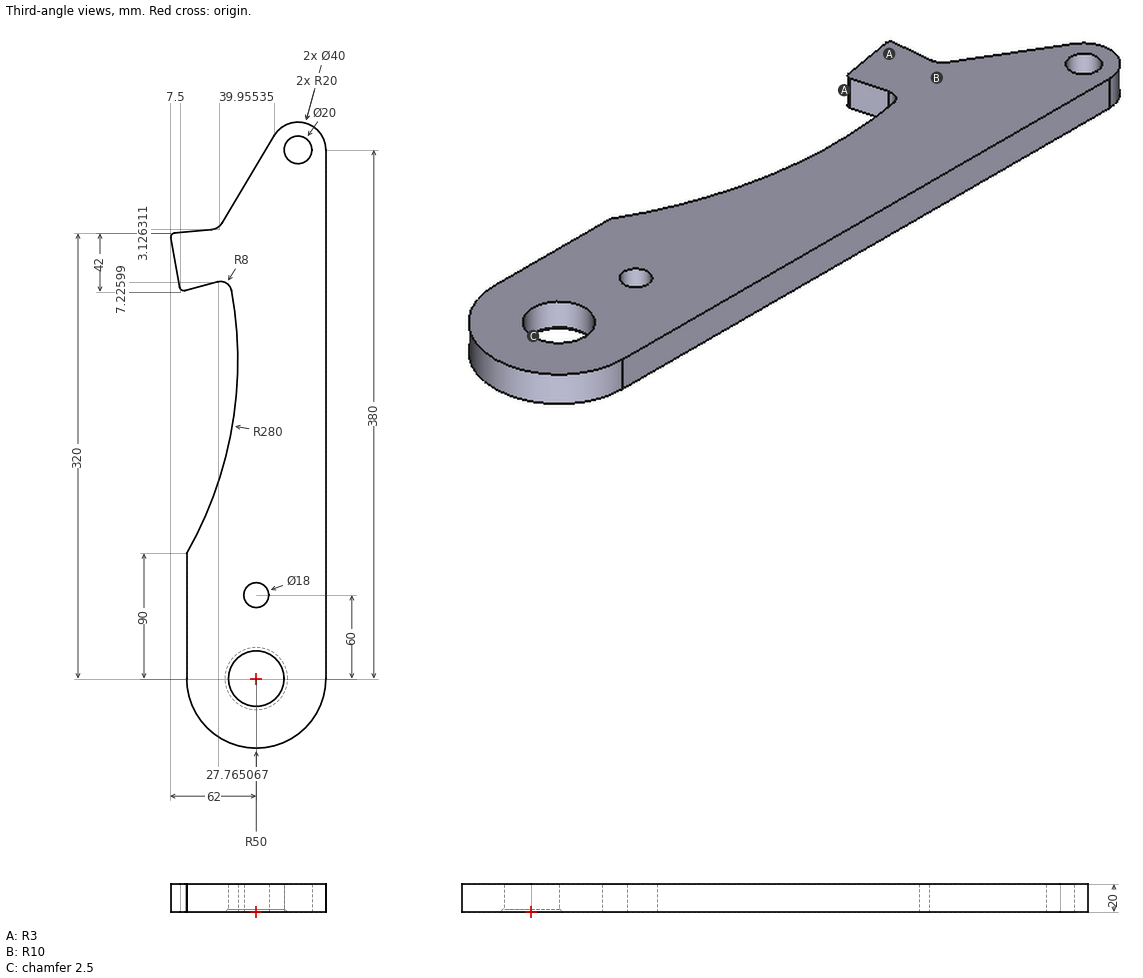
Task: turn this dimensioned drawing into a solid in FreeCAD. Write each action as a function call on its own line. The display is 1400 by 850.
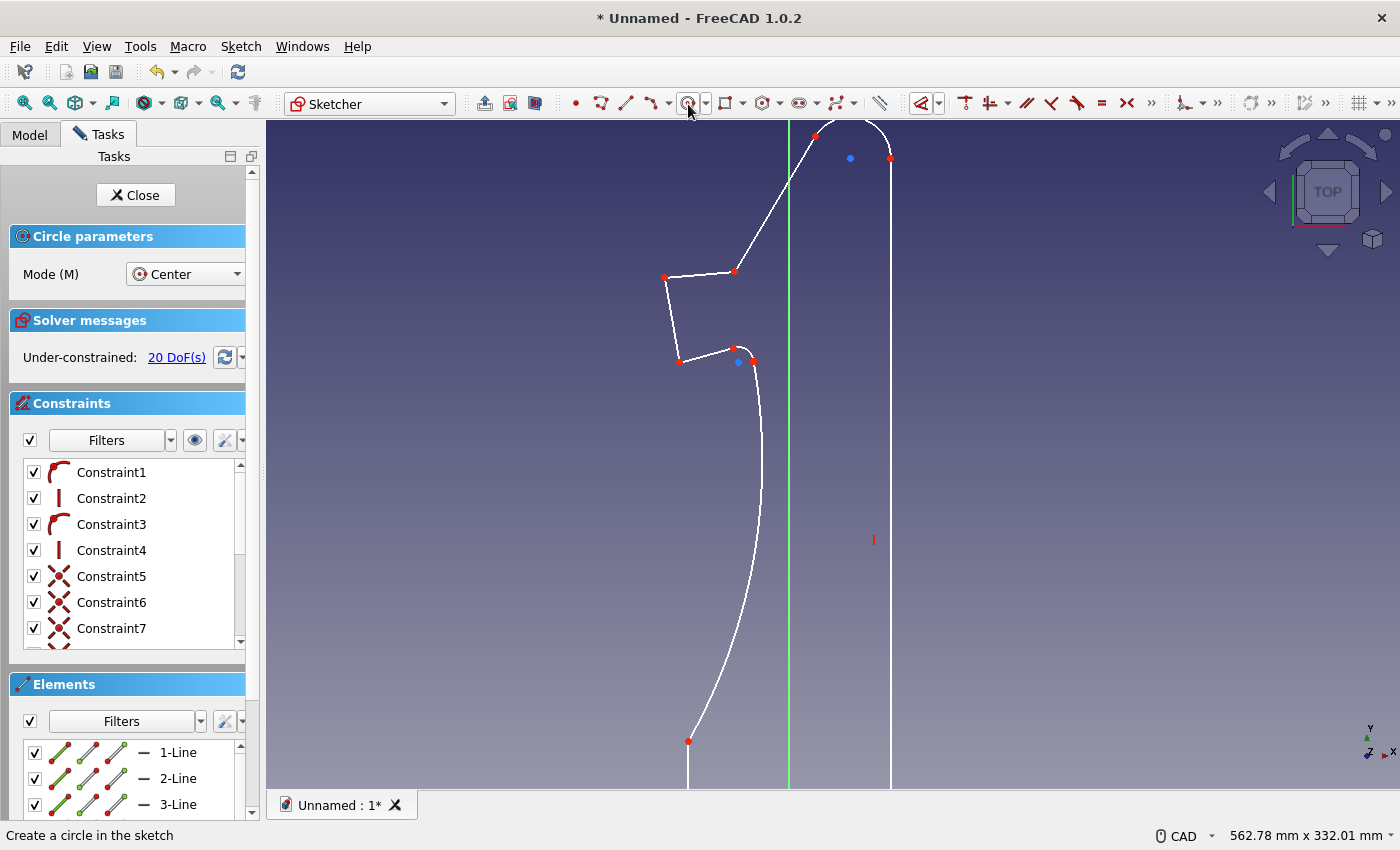
scroll(754, 360, down, 4)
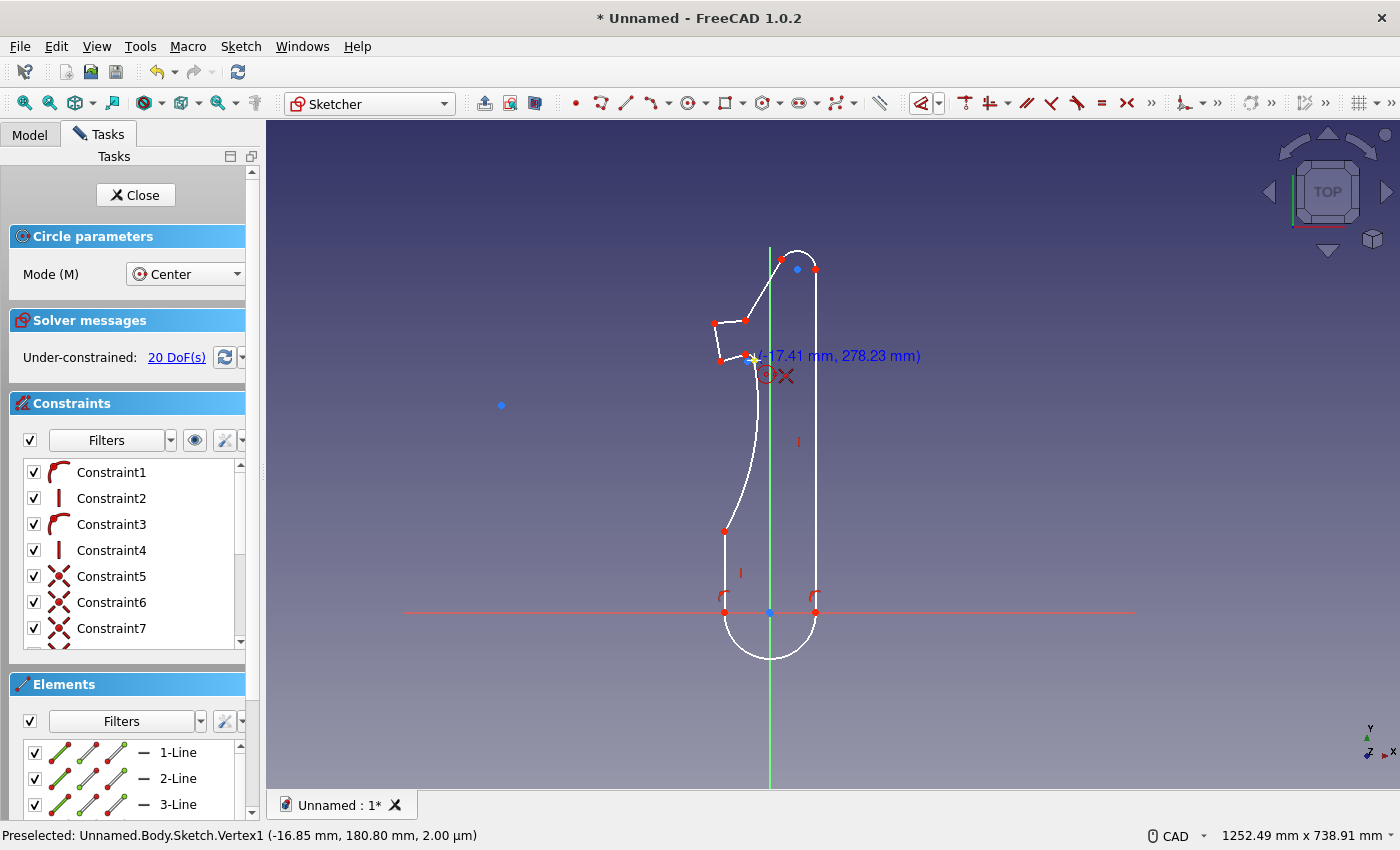
scroll(770, 613, up, 2)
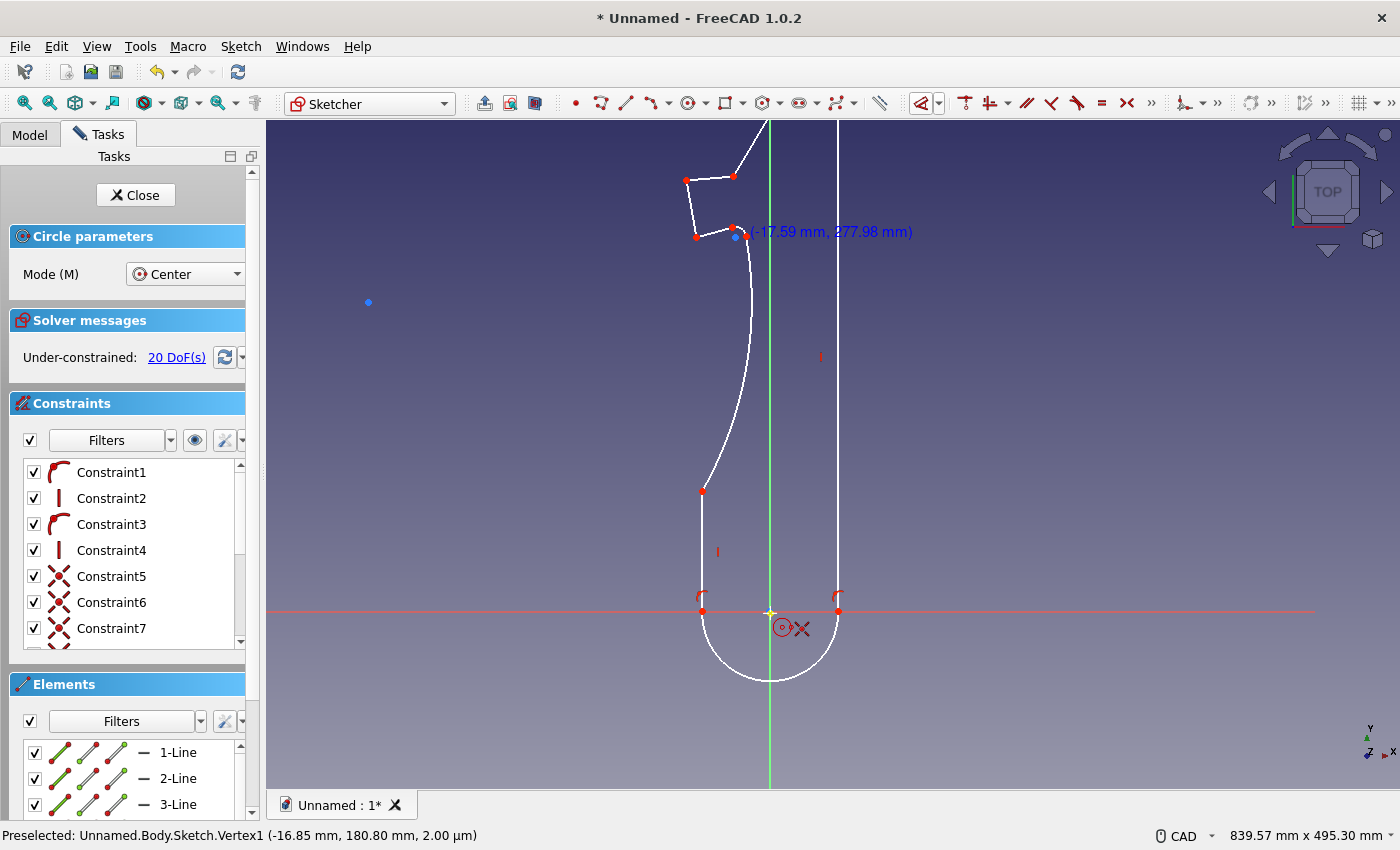
click(770, 612)
move(789, 593)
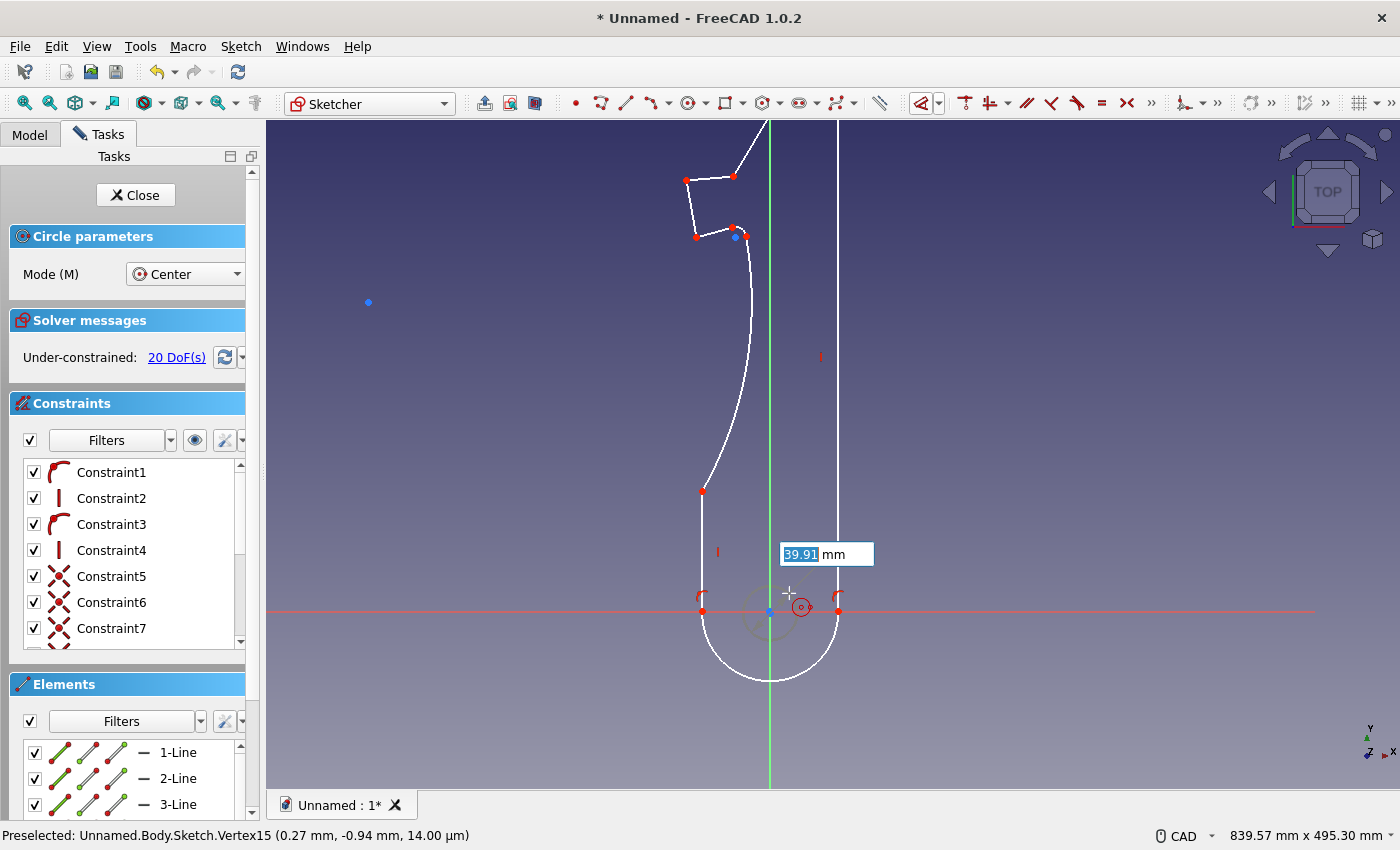
text(40)
key(Return)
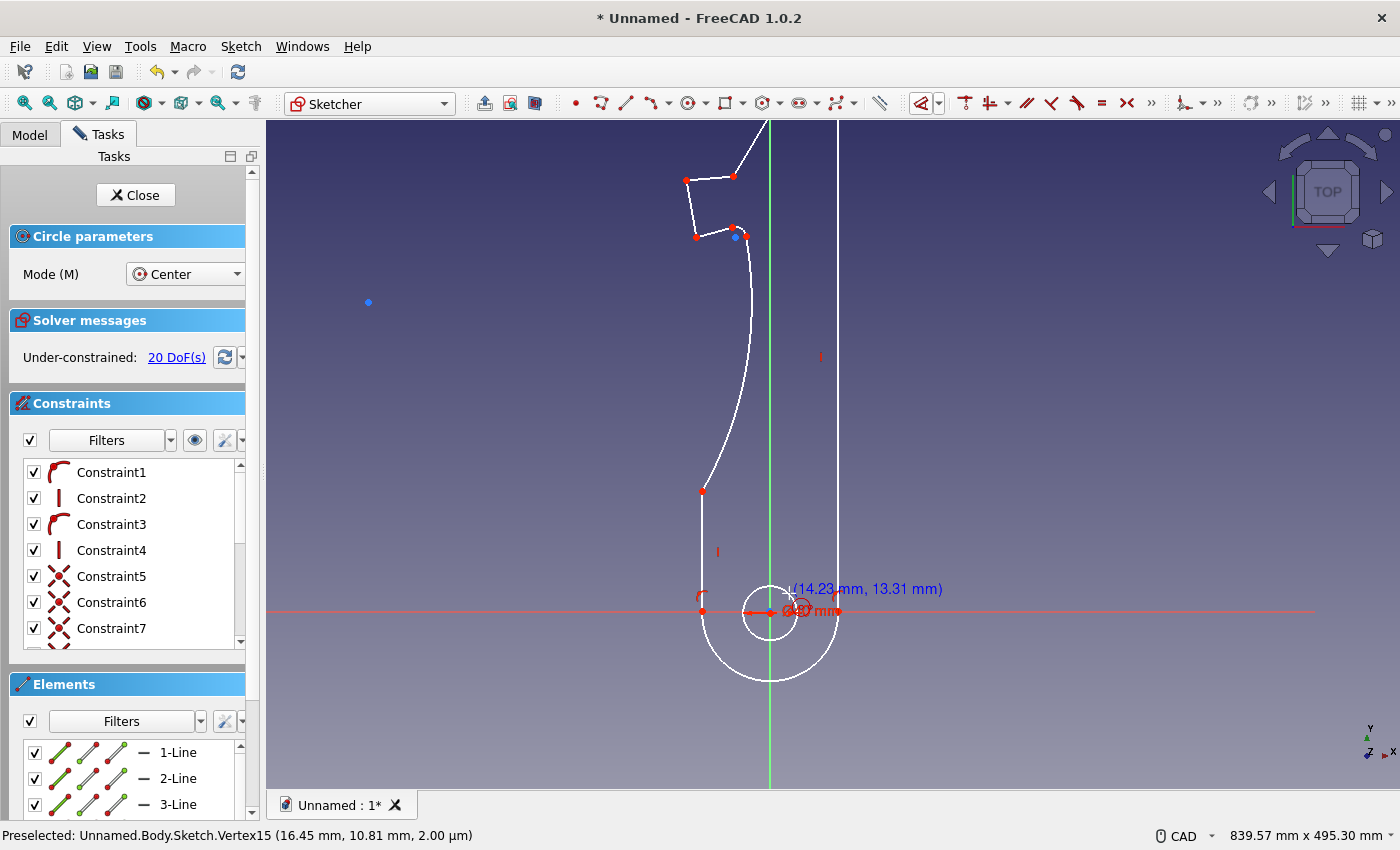
scroll(770, 531, up, 4)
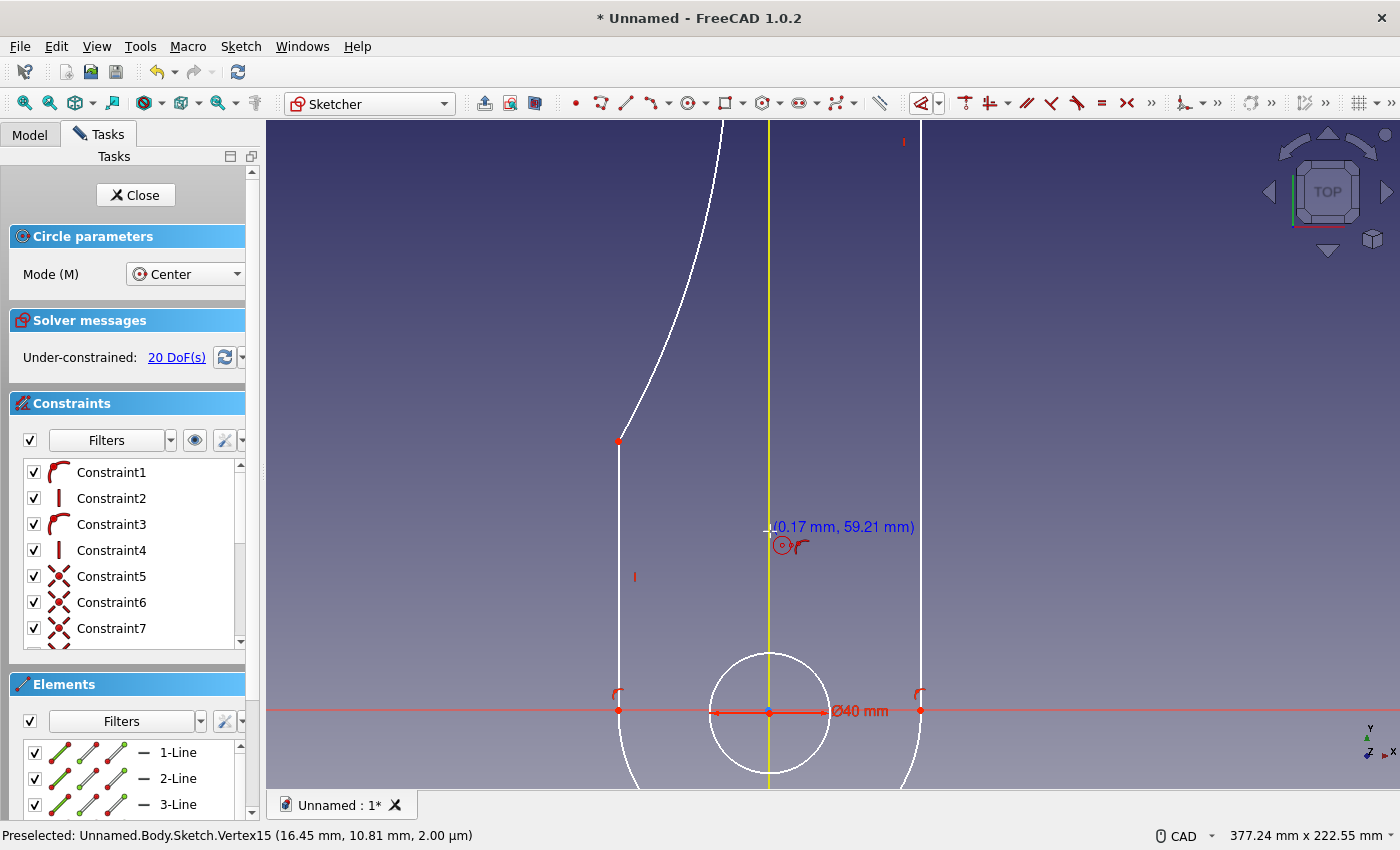
click(769, 530)
move(788, 511)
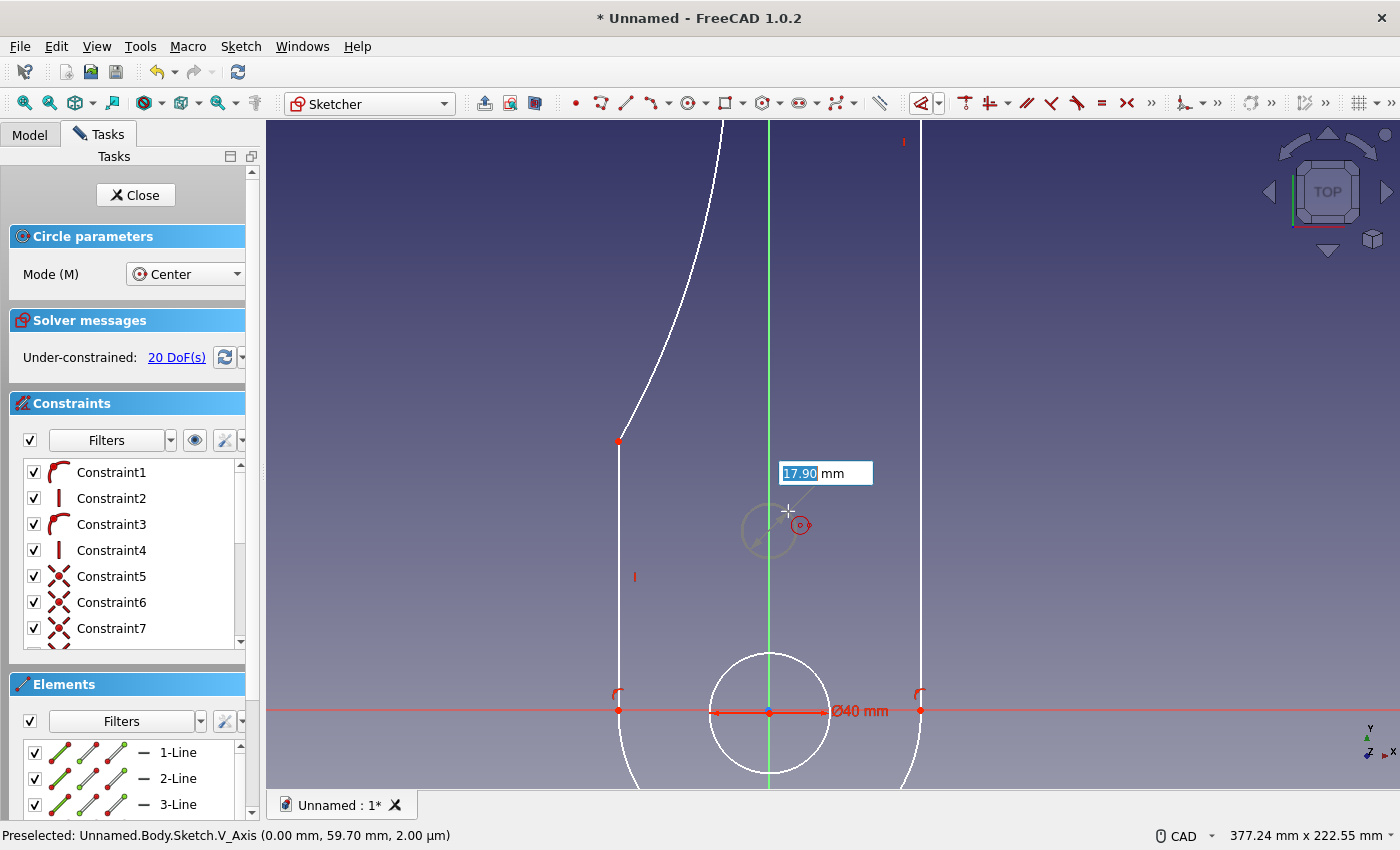
text(18)
key(Return)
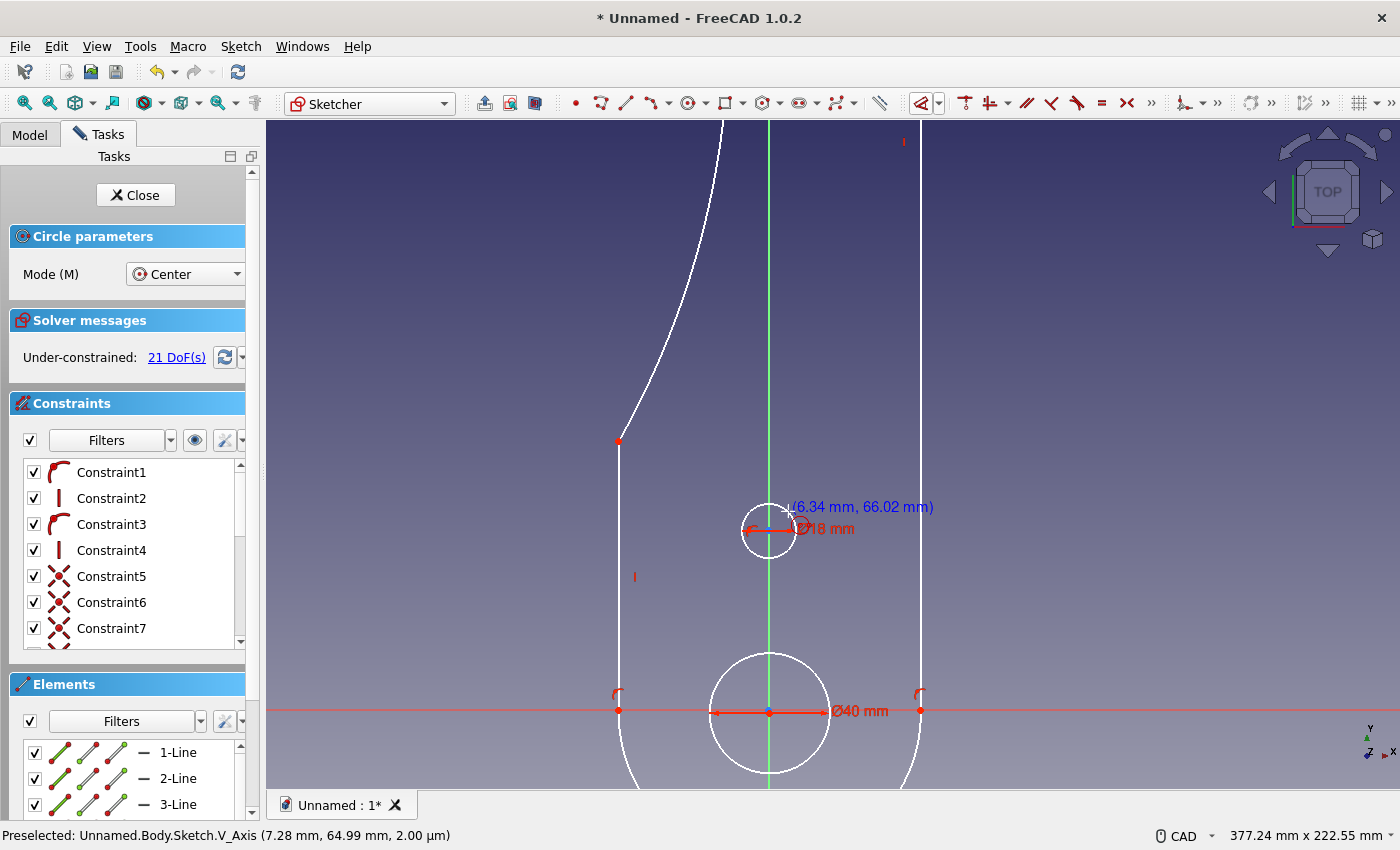
scroll(770, 570, down, 6)